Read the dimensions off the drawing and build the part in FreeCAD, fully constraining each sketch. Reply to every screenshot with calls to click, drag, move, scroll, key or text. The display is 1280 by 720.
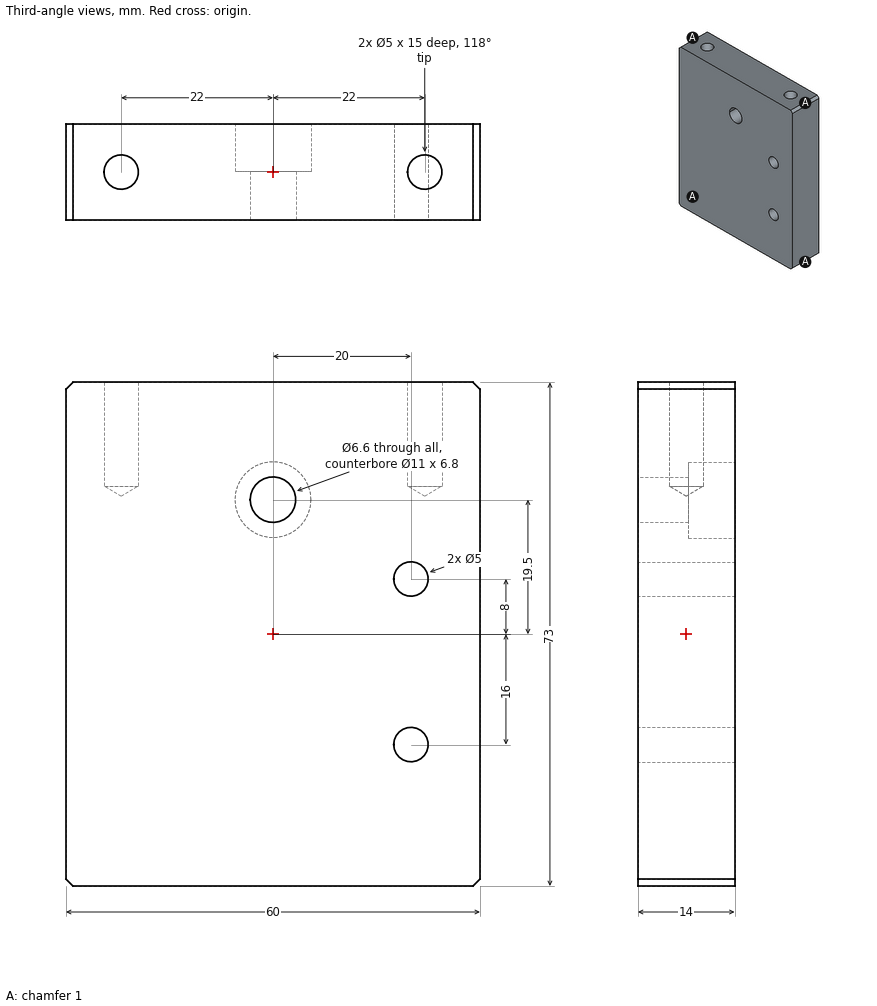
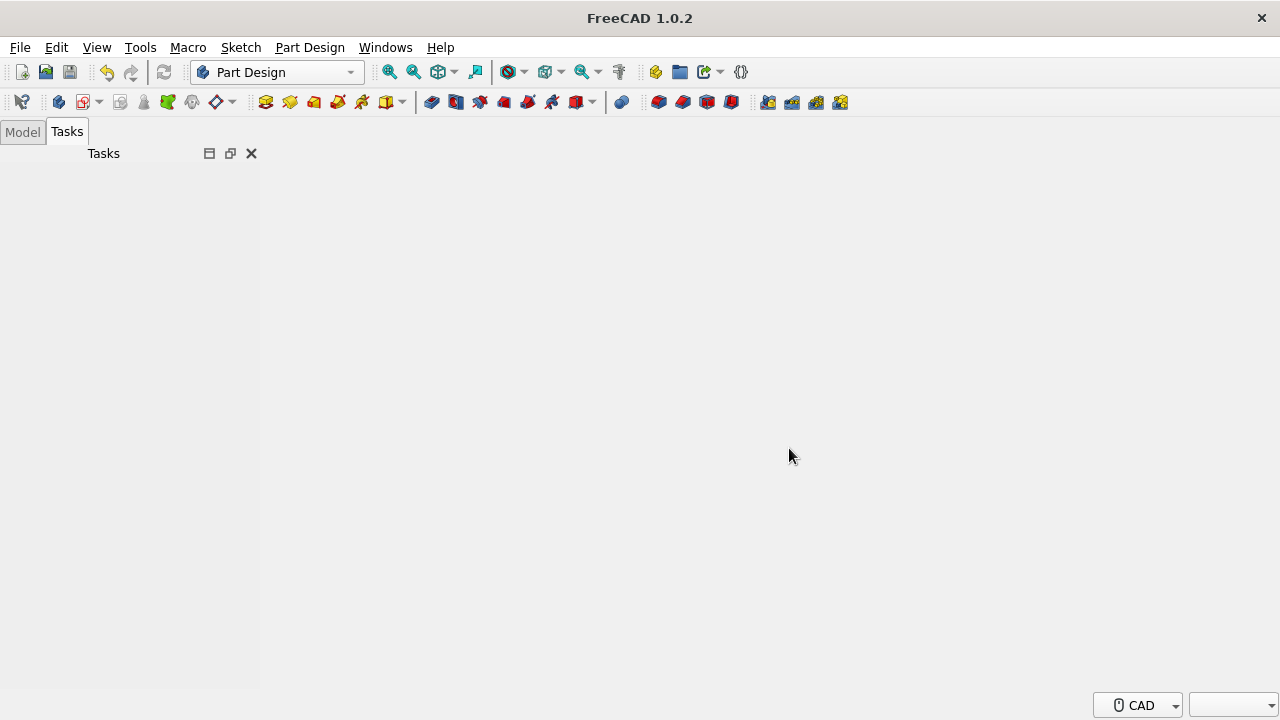
click(22, 72)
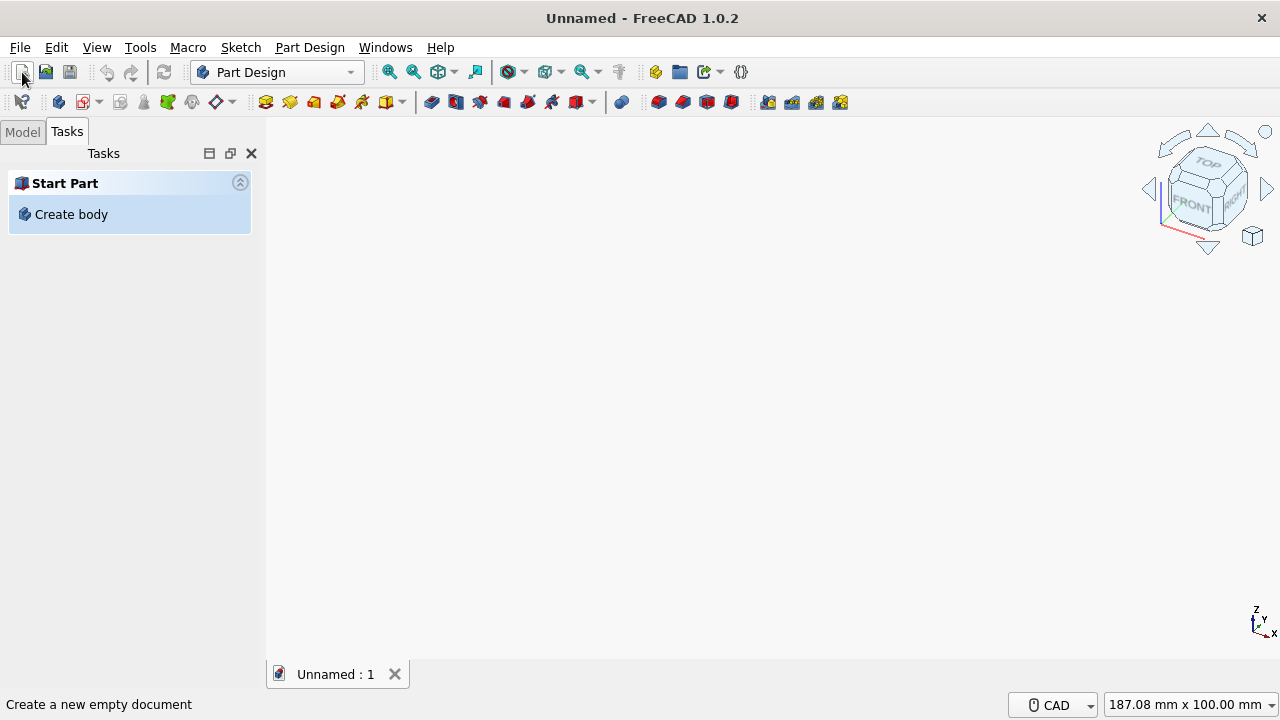
click(84, 102)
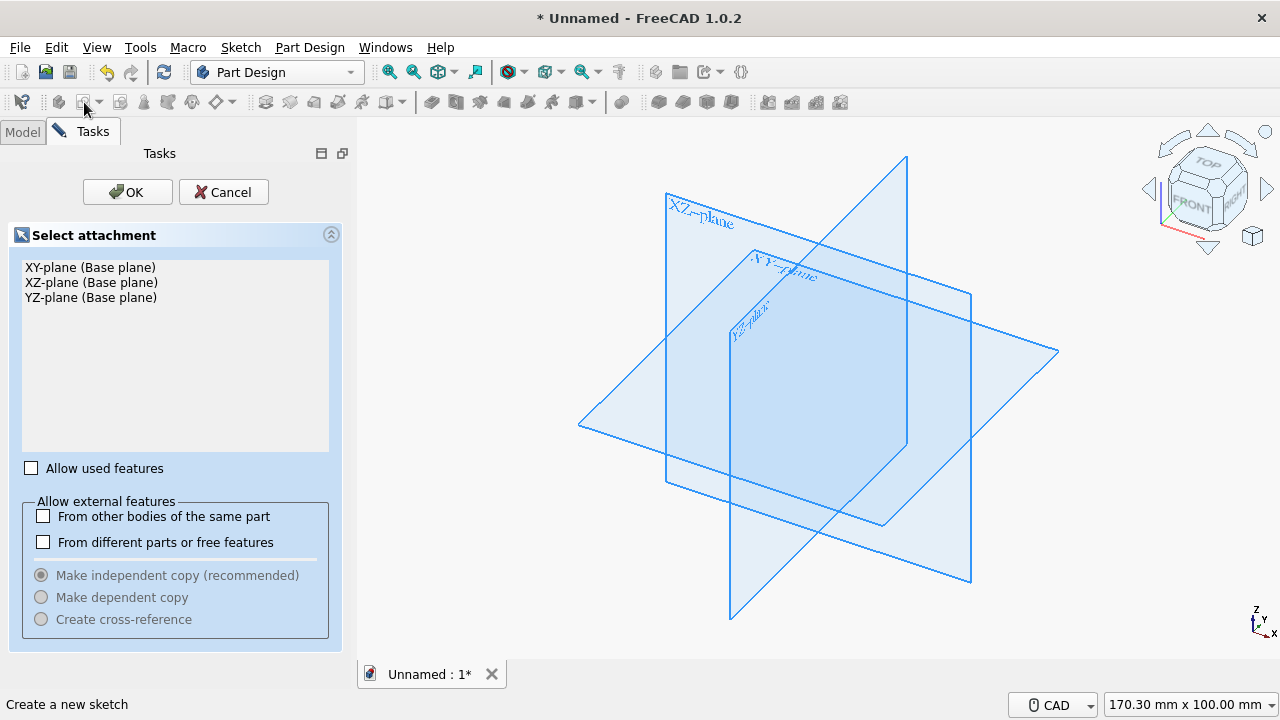
click(82, 282)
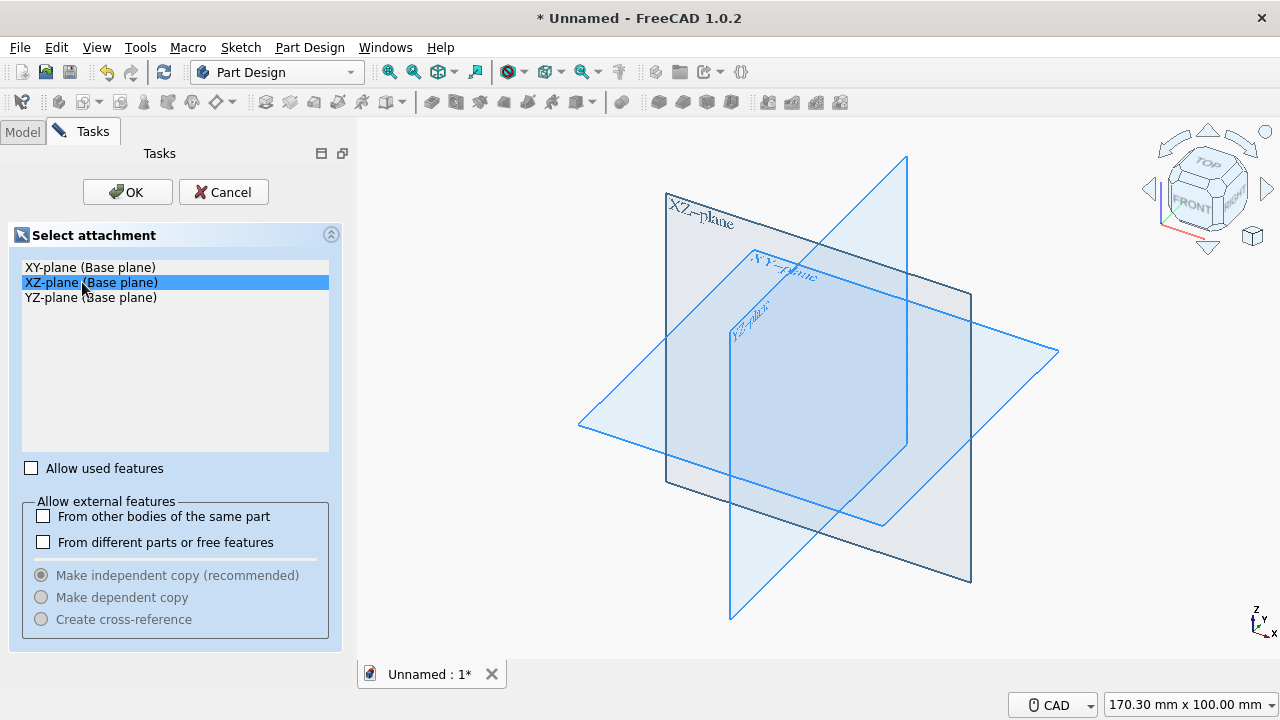
click(128, 192)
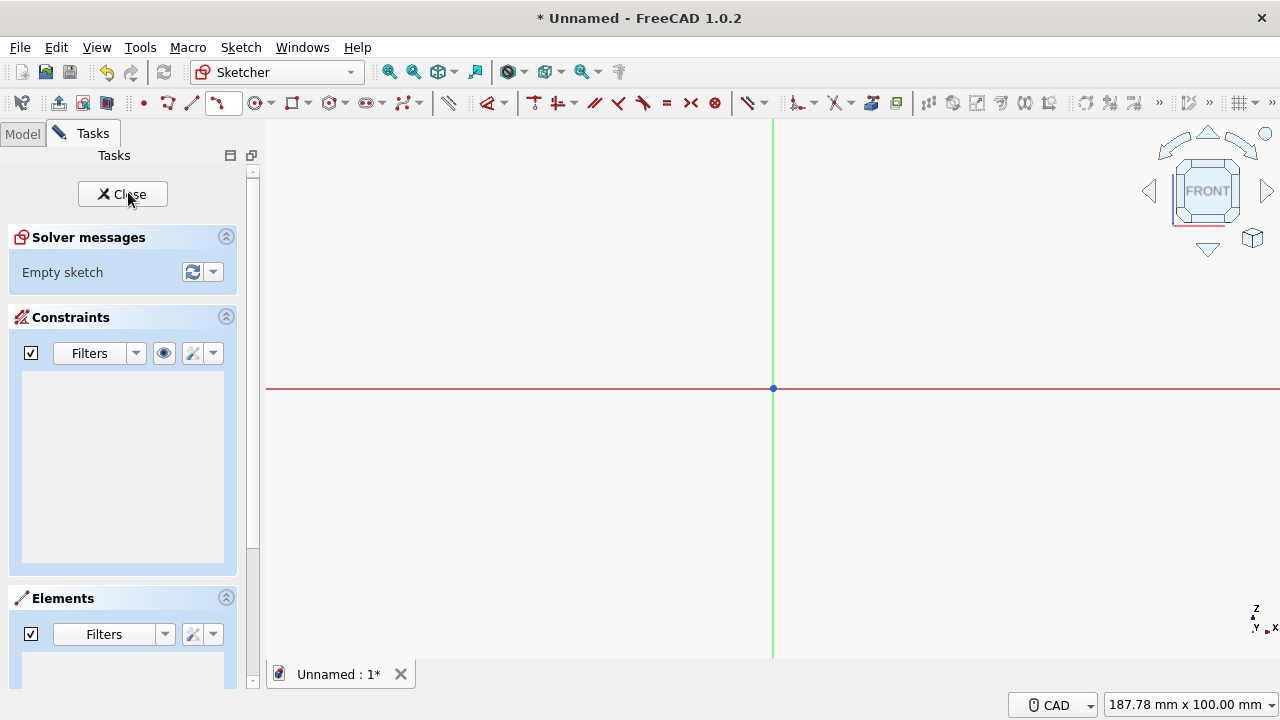
click(310, 104)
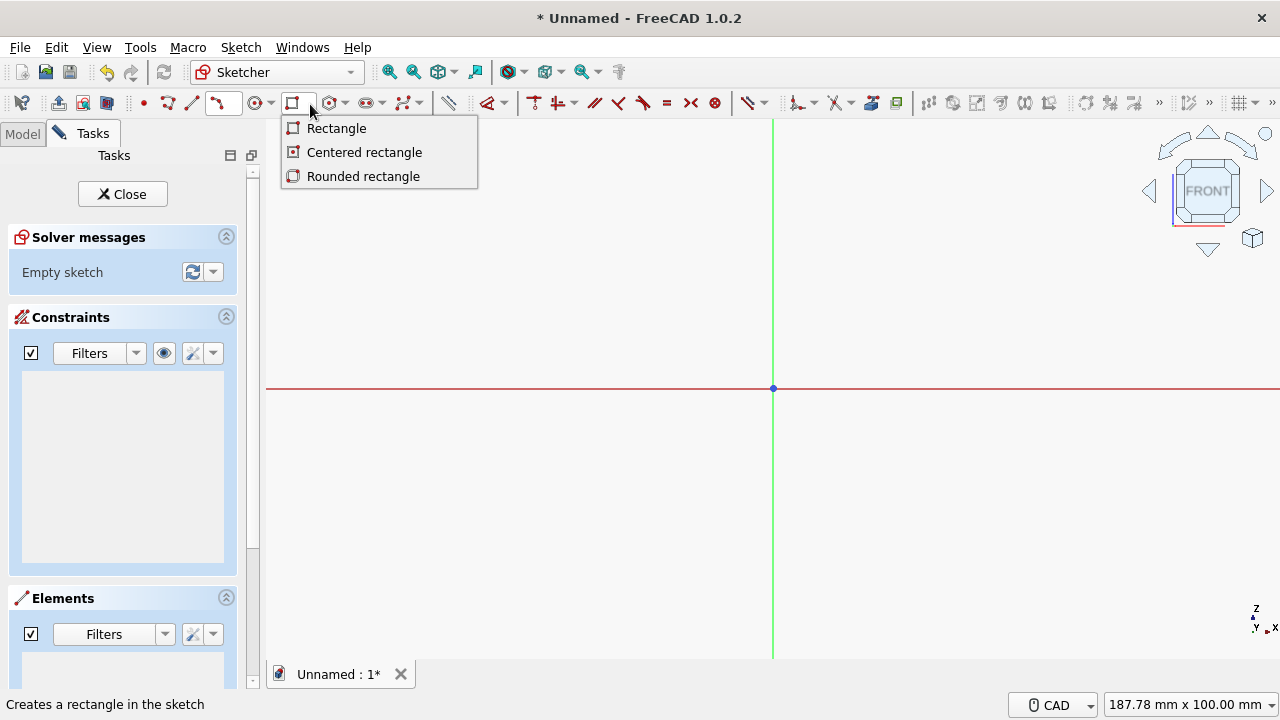
click(380, 152)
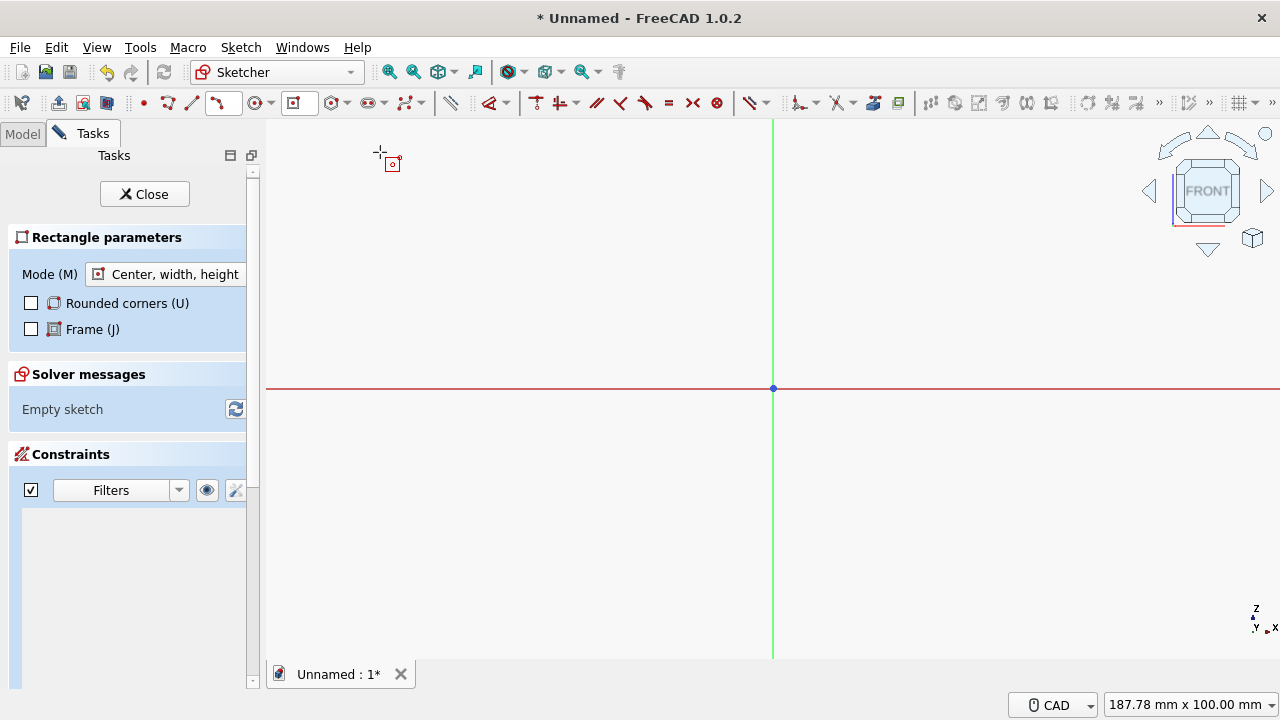
click(773, 389)
click(935, 192)
key(Escape)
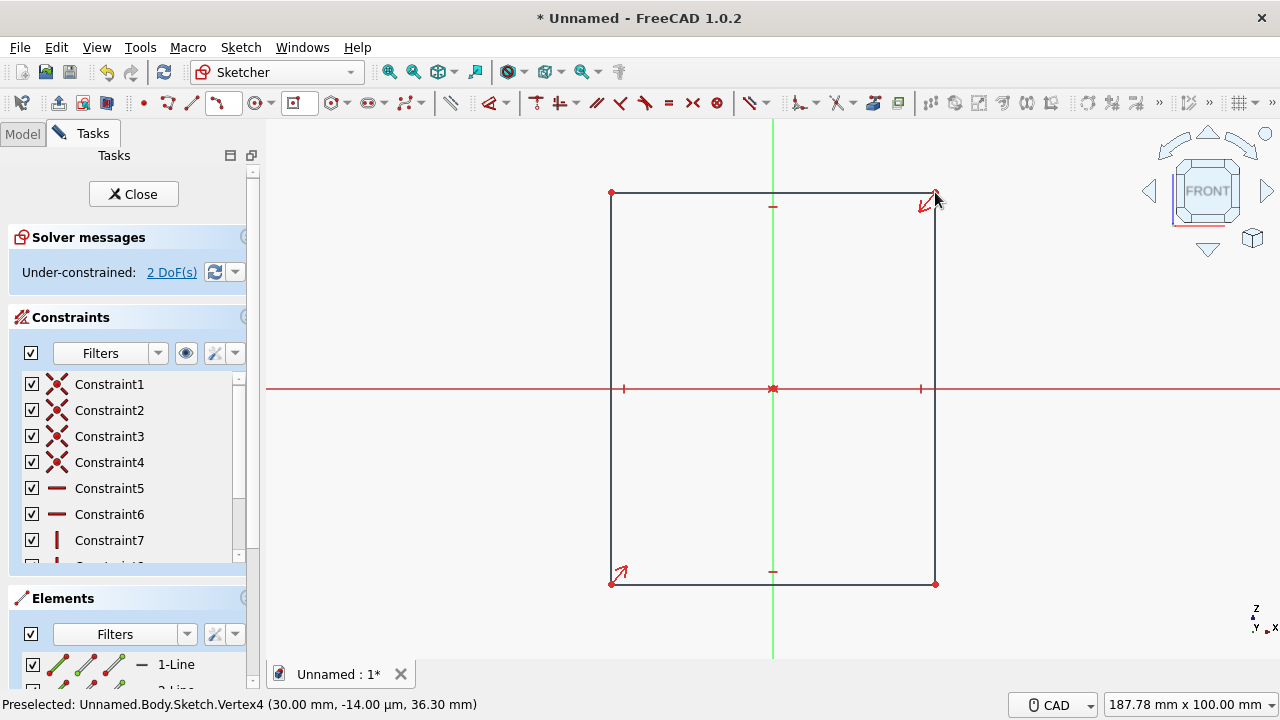
click(490, 104)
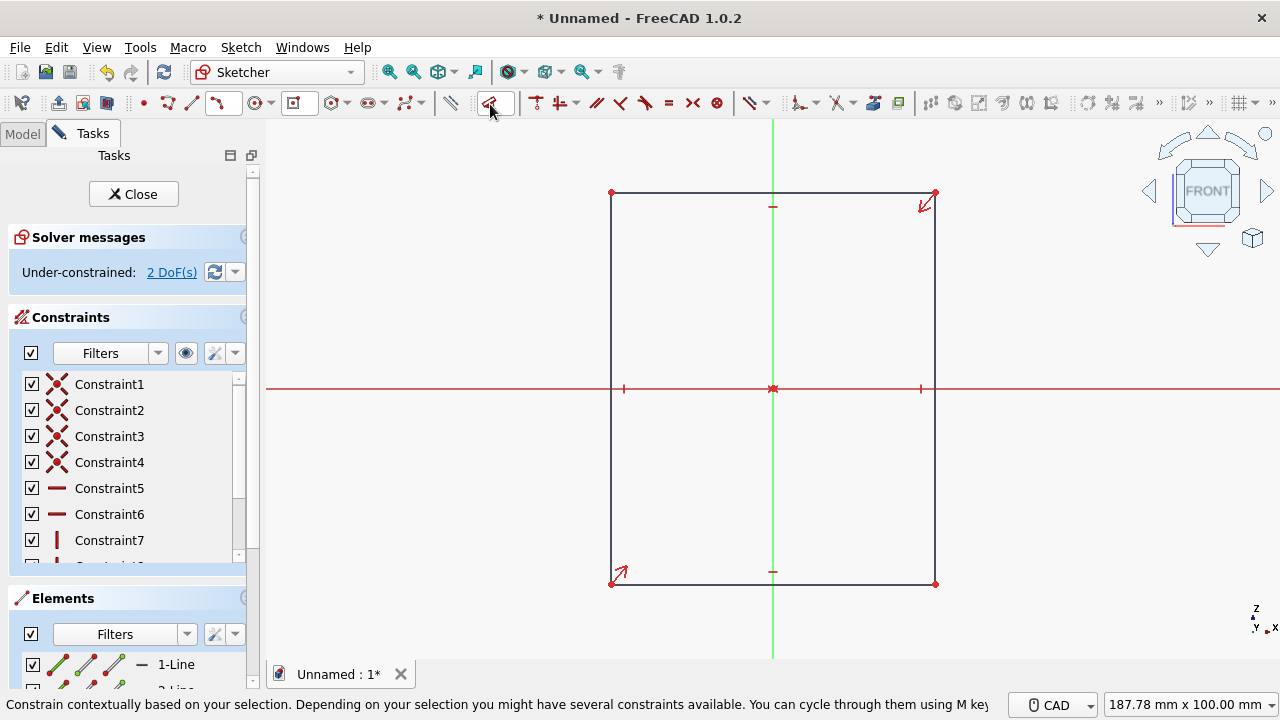
click(708, 585)
click(698, 619)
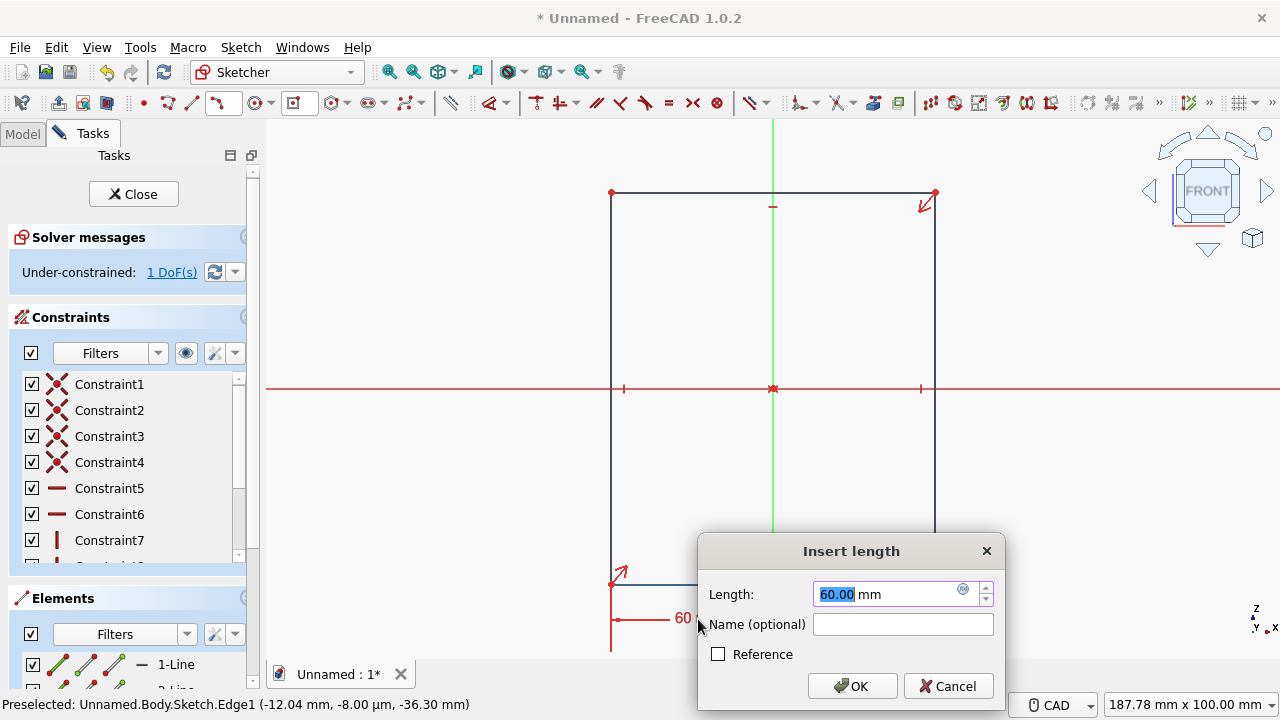
text(60)
key(Return)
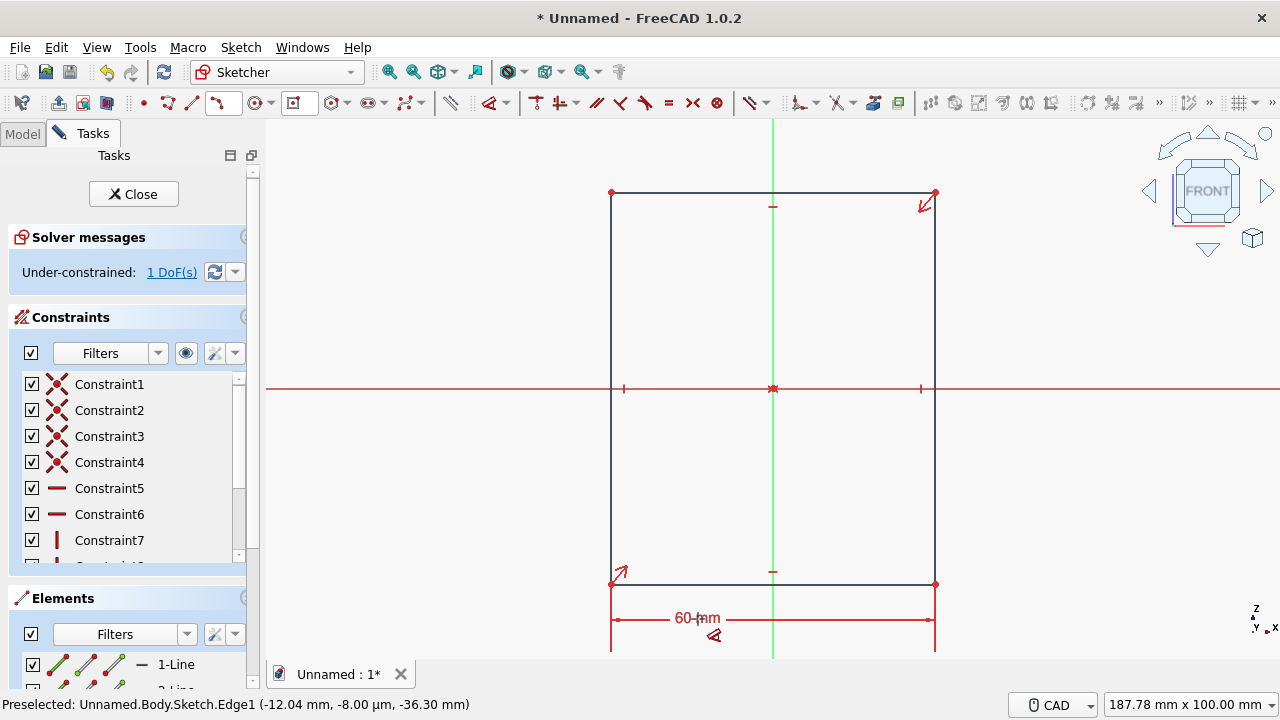
click(935, 467)
click(969, 299)